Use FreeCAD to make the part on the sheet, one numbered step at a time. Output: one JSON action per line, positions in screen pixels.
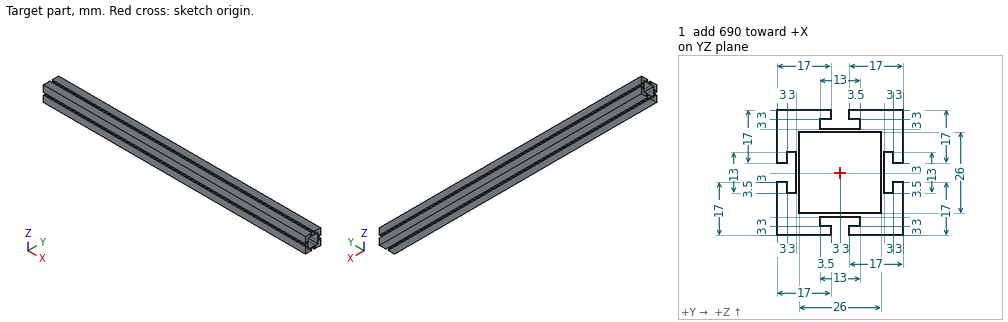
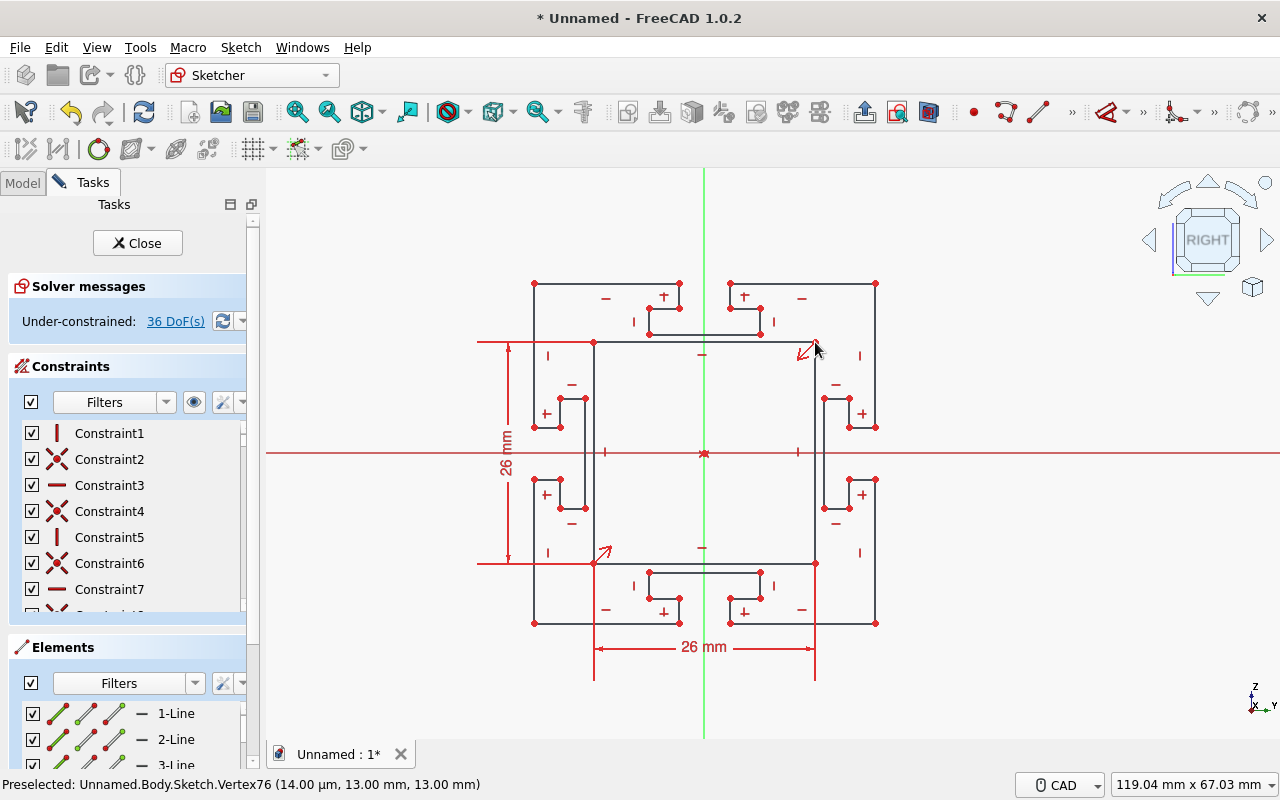
{"action": "key", "text": "d"}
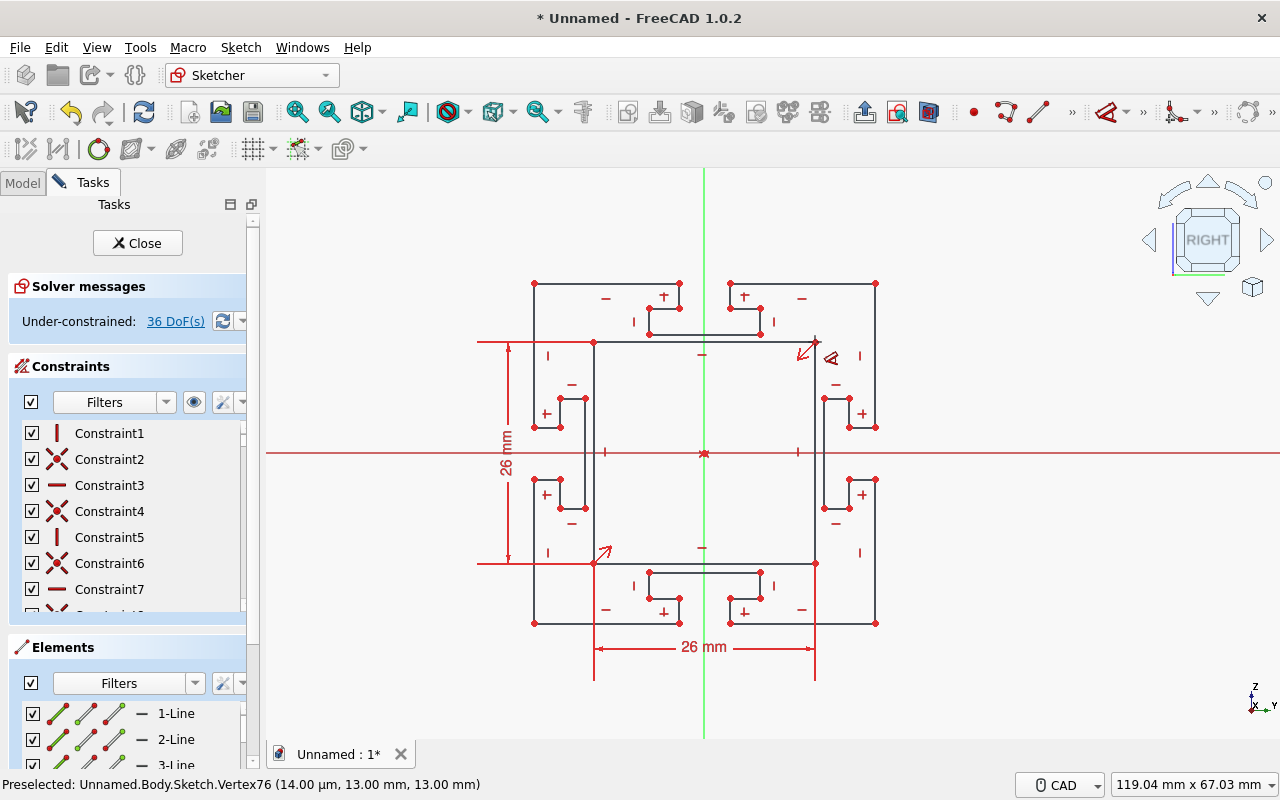
{"action": "scroll", "coordinate": [575, 509], "scroll_direction": "up", "scroll_amount": 3}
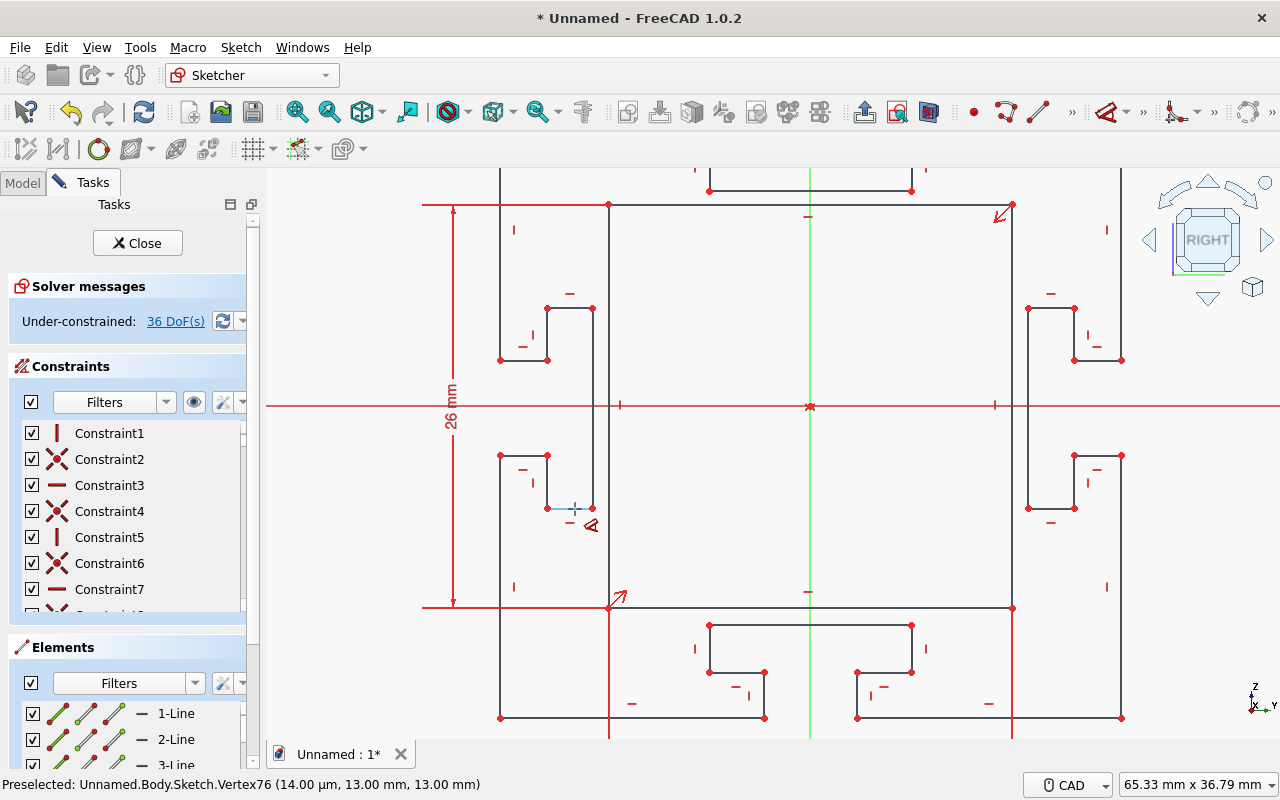
{"action": "left_click", "coordinate": [575, 509]}
{"action": "left_click", "coordinate": [570, 543]}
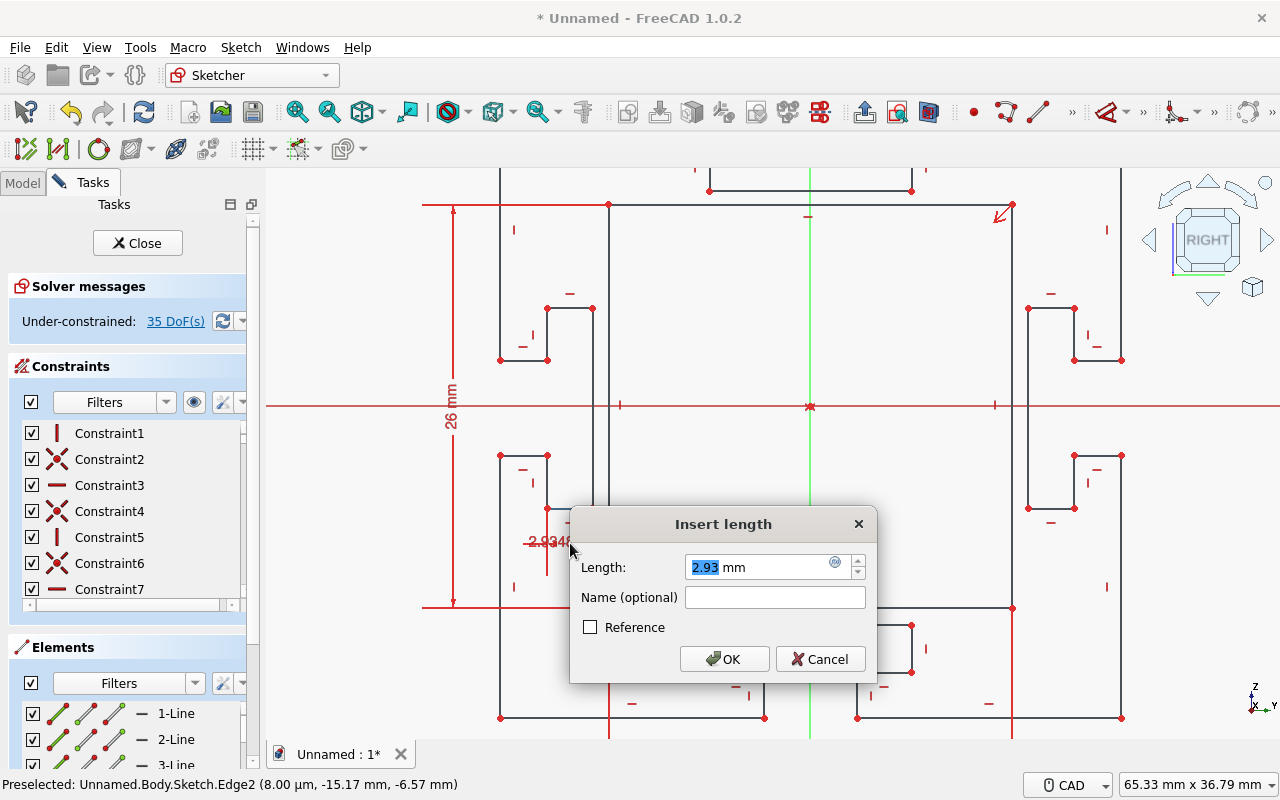
{"action": "type", "text": "3"}
{"action": "key", "text": "Return"}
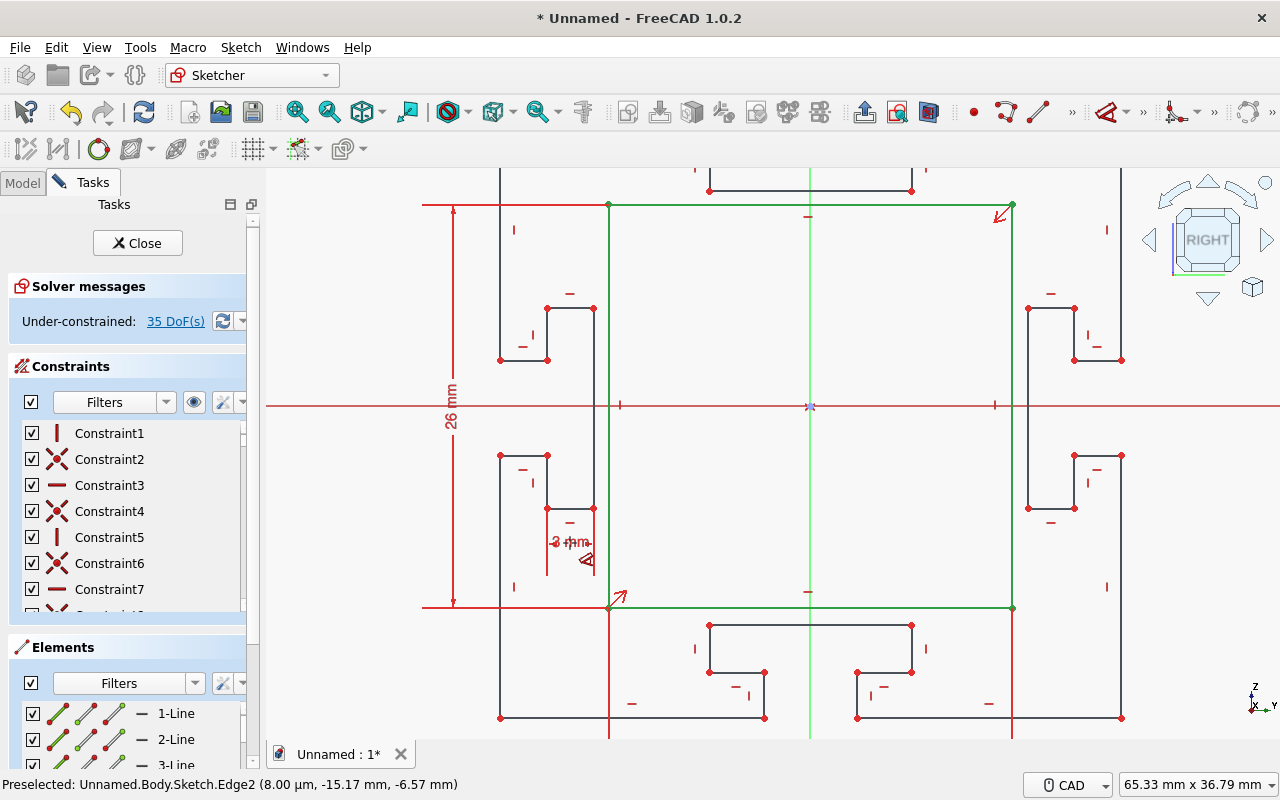
{"action": "left_click", "coordinate": [533, 456]}
{"action": "left_click", "coordinate": [524, 490]}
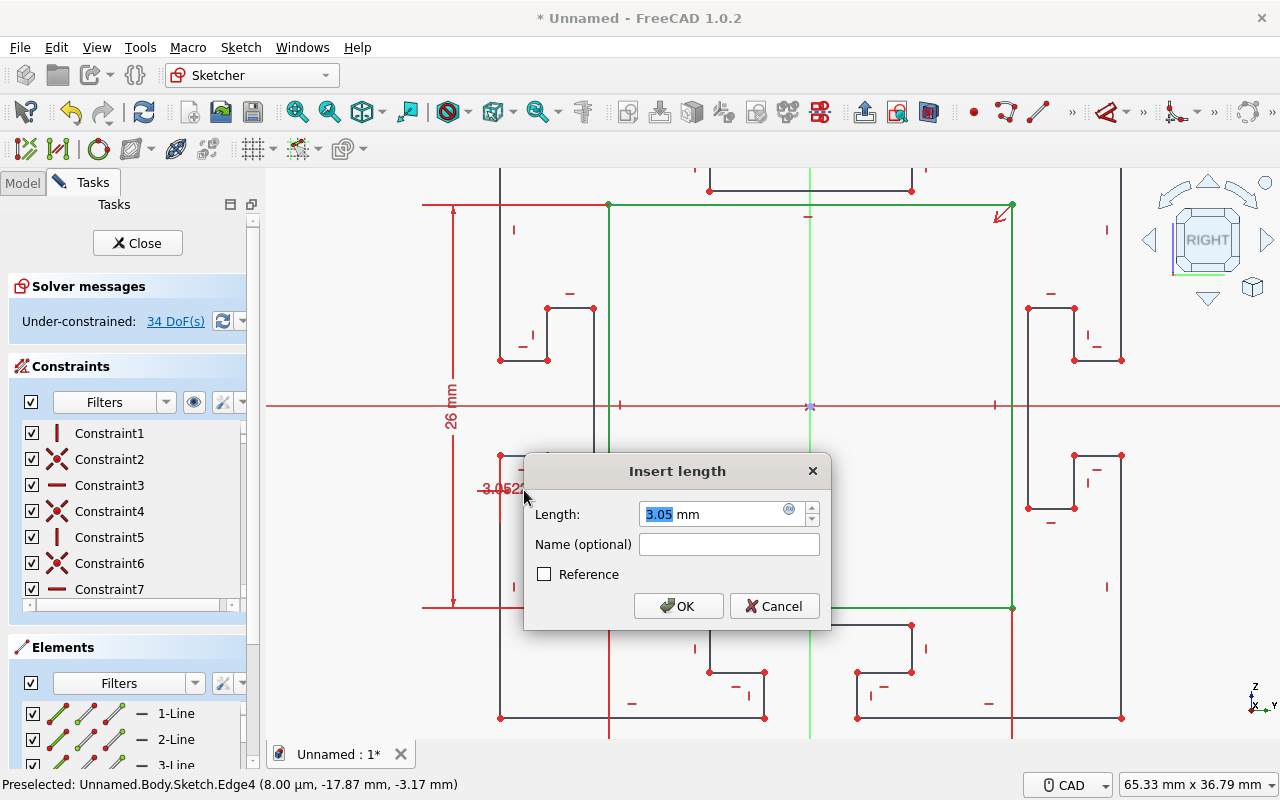
{"action": "type", "text": "3"}
{"action": "key", "text": "Return"}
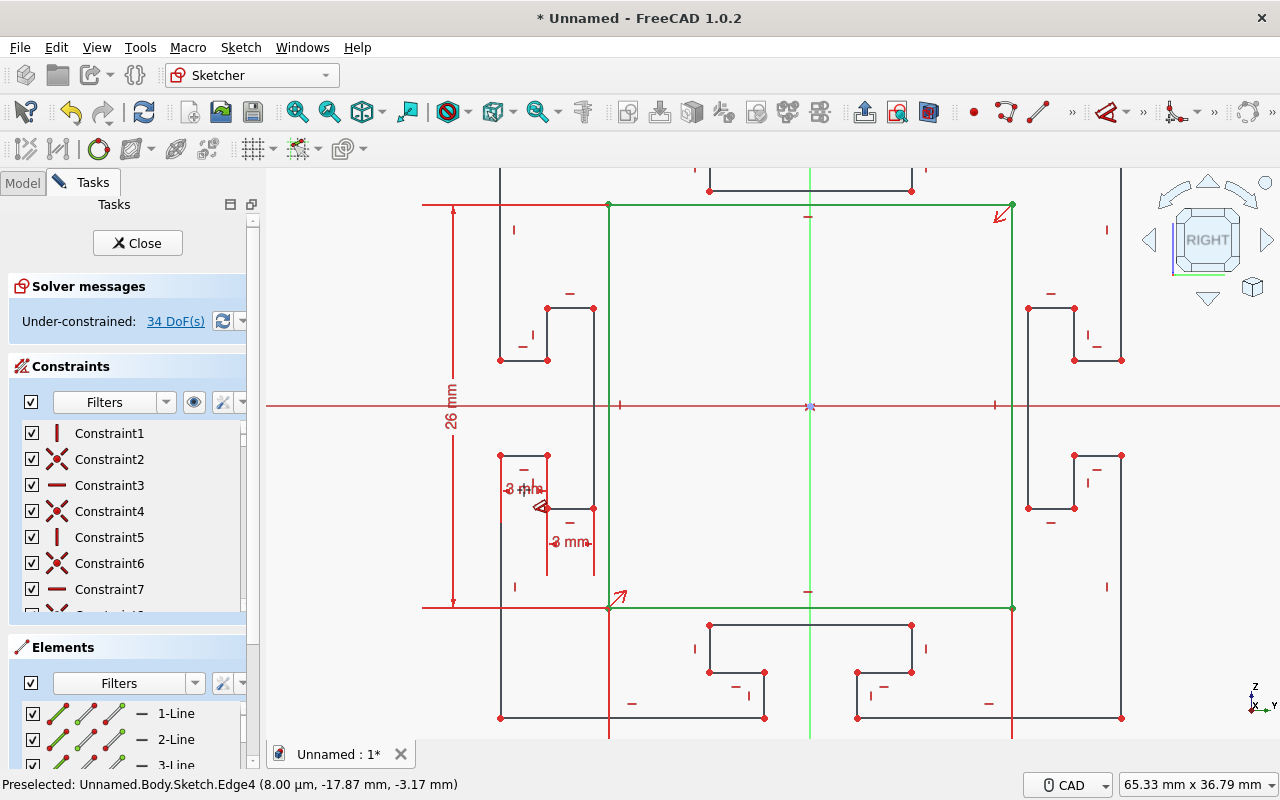
{"action": "left_click", "coordinate": [764, 704]}
{"action": "left_click", "coordinate": [730, 692]}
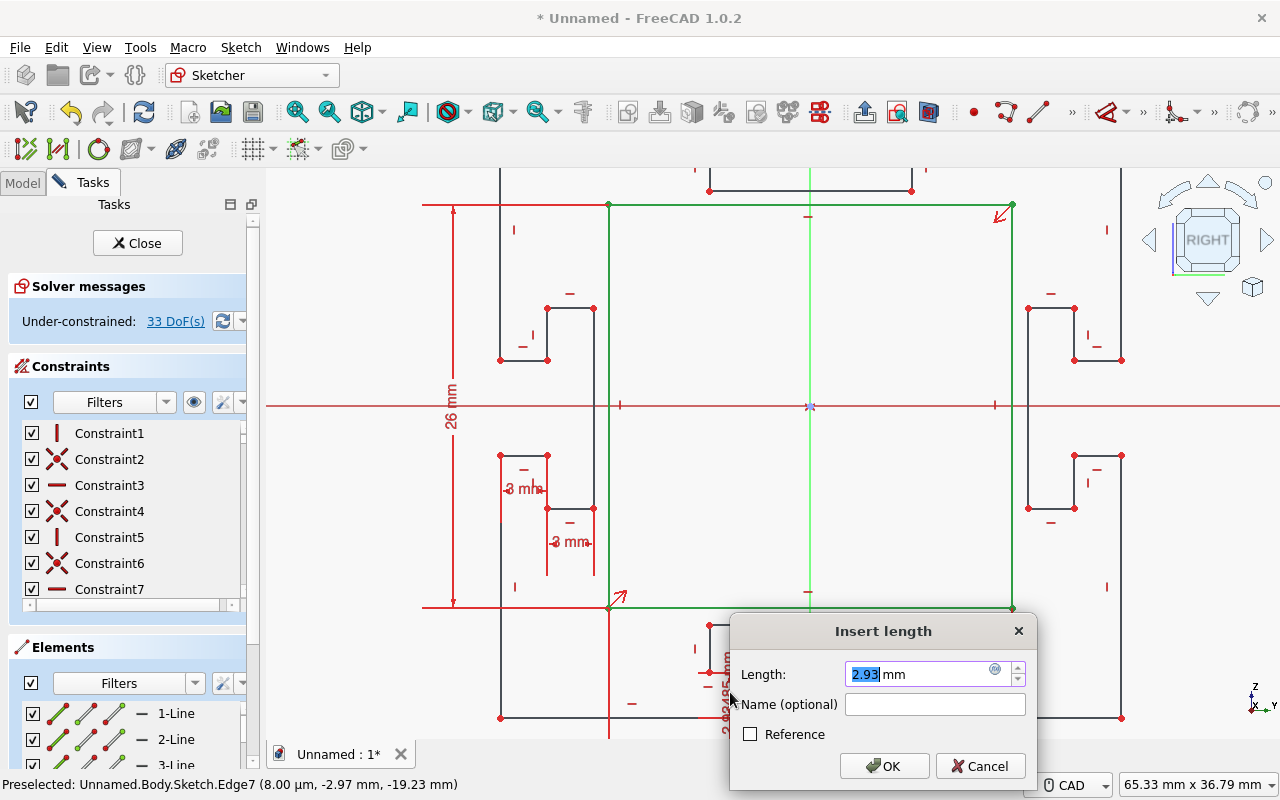
{"action": "type", "text": "3"}
{"action": "key", "text": "Return"}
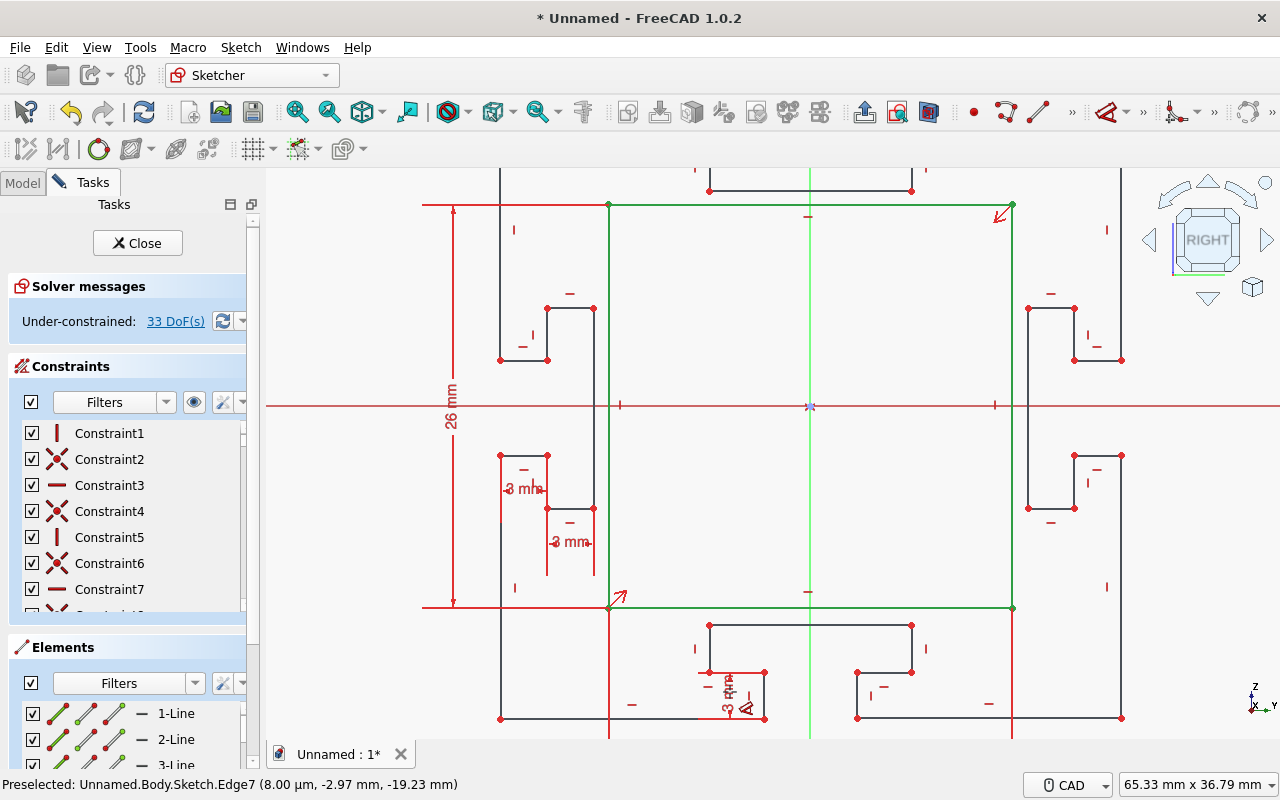
{"action": "left_click", "coordinate": [710, 658]}
{"action": "left_click", "coordinate": [676, 649]}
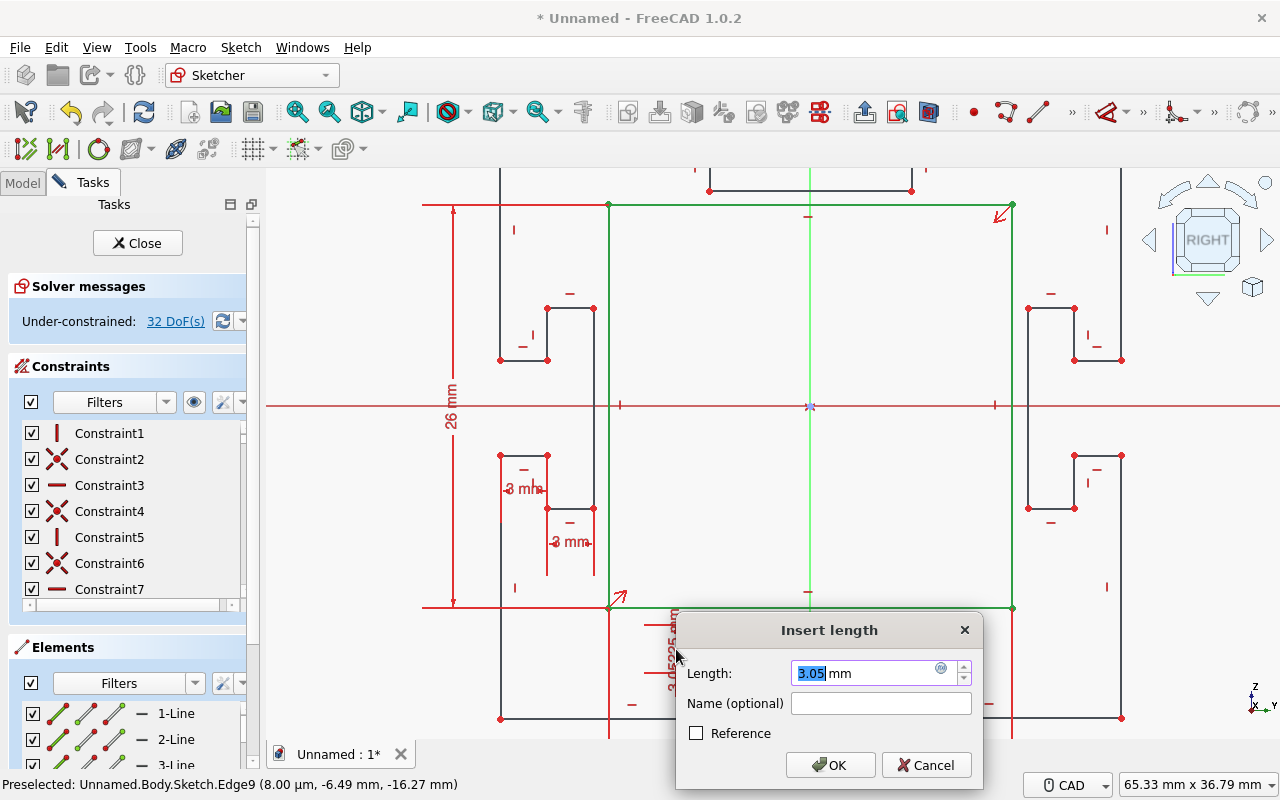
{"action": "type", "text": "3"}
{"action": "key", "text": "Return"}